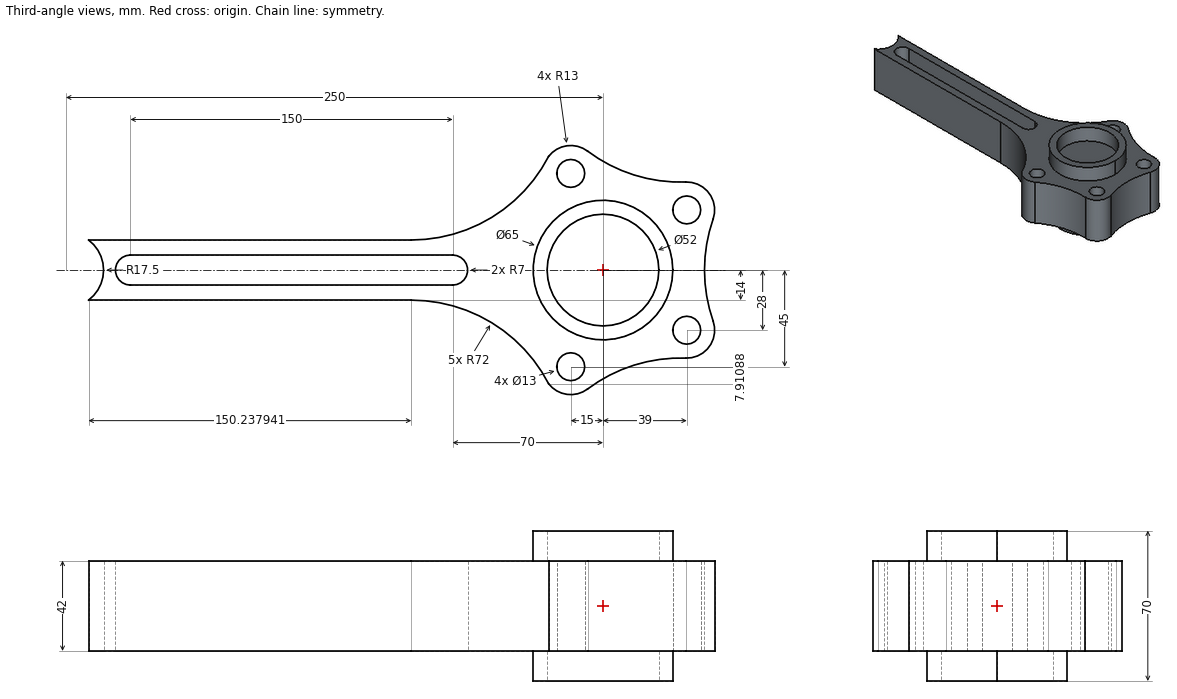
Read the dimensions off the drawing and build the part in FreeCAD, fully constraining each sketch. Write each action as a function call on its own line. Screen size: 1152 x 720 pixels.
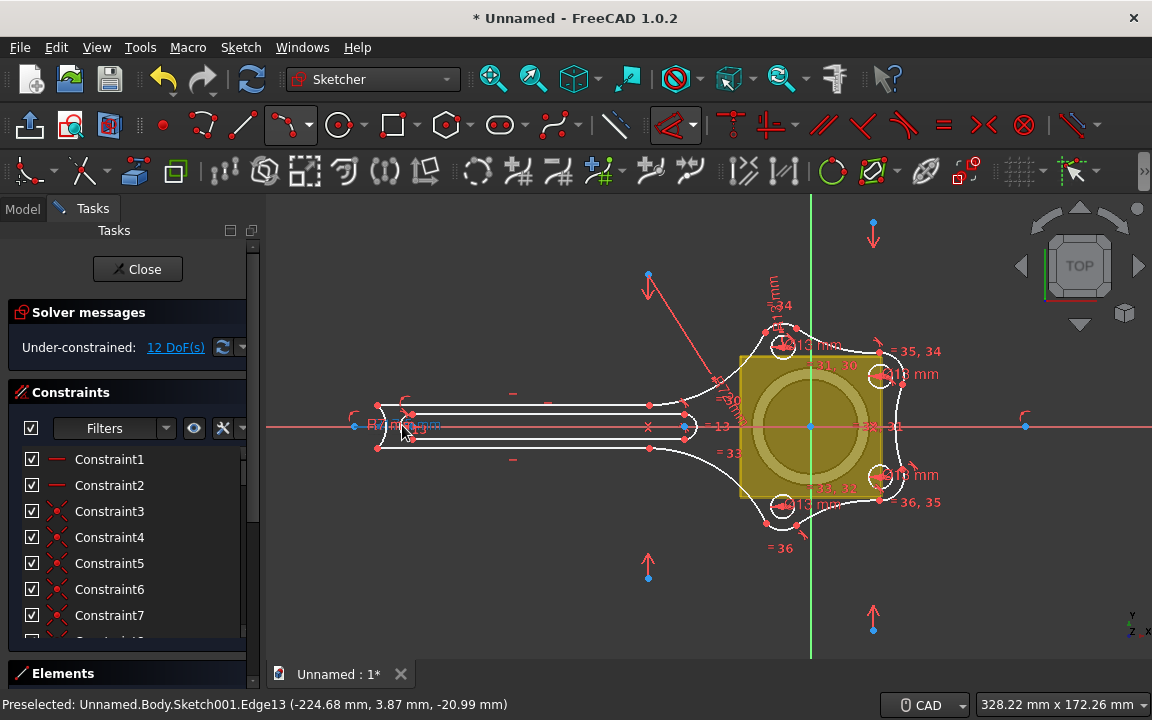
scroll(783, 507, up, 2)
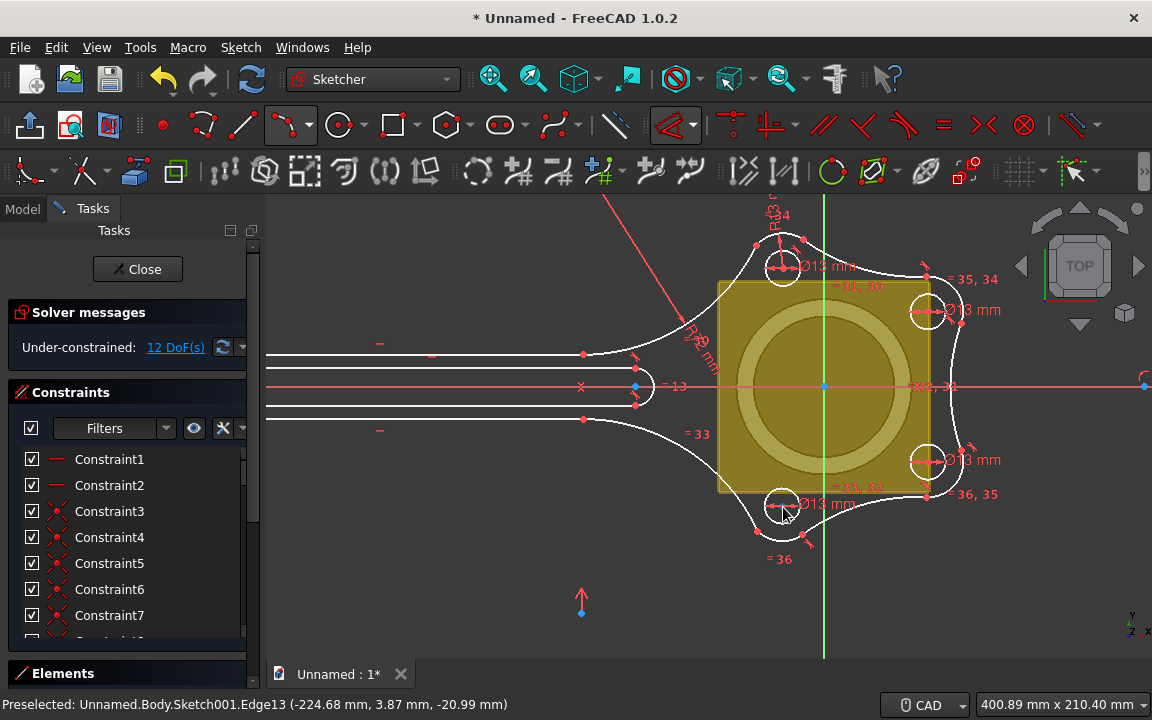
click(782, 506)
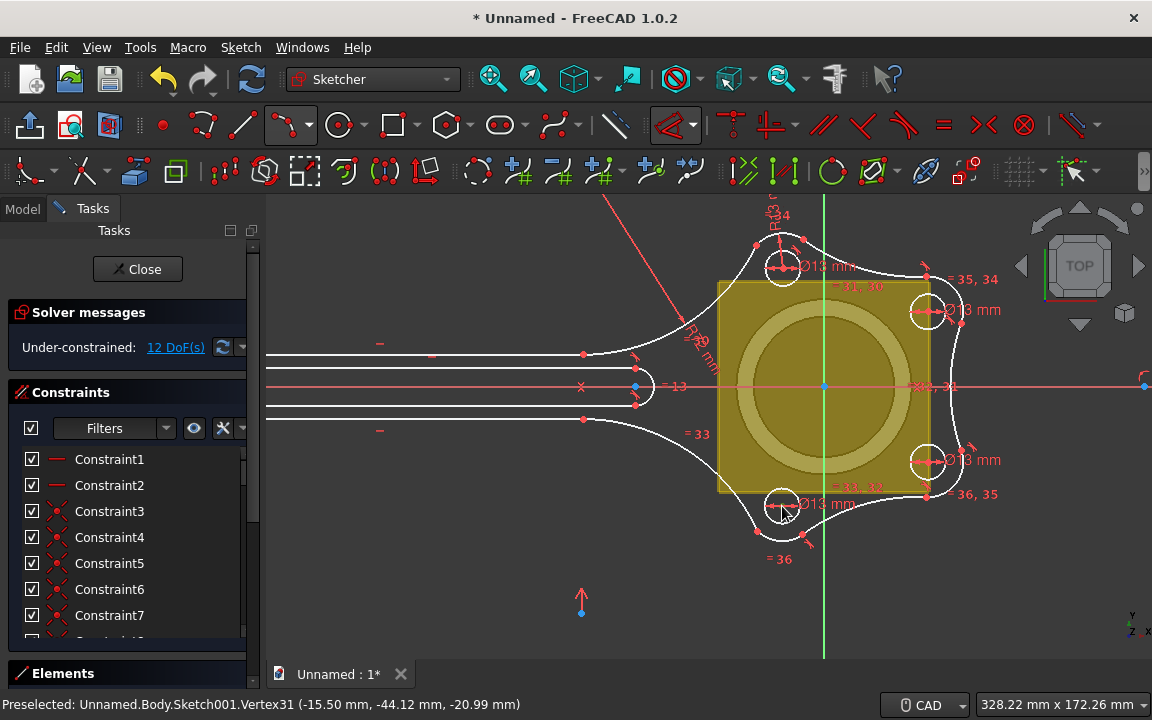
key(l)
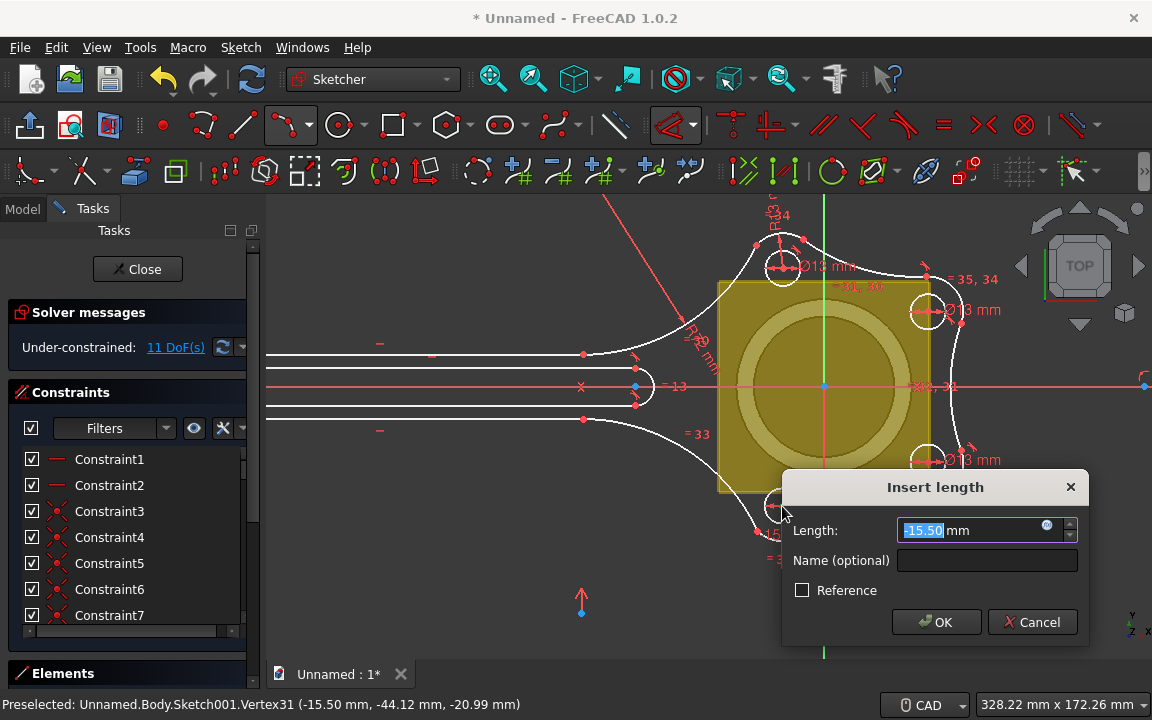
text(-15)
key(Return)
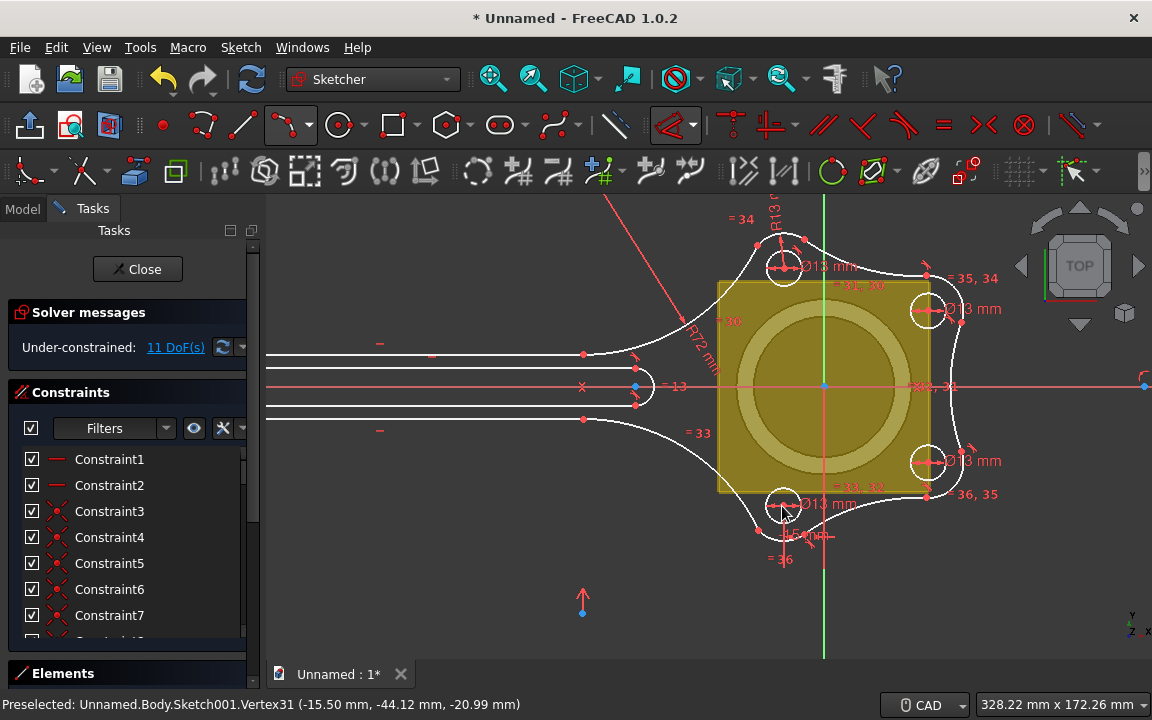
click(784, 506)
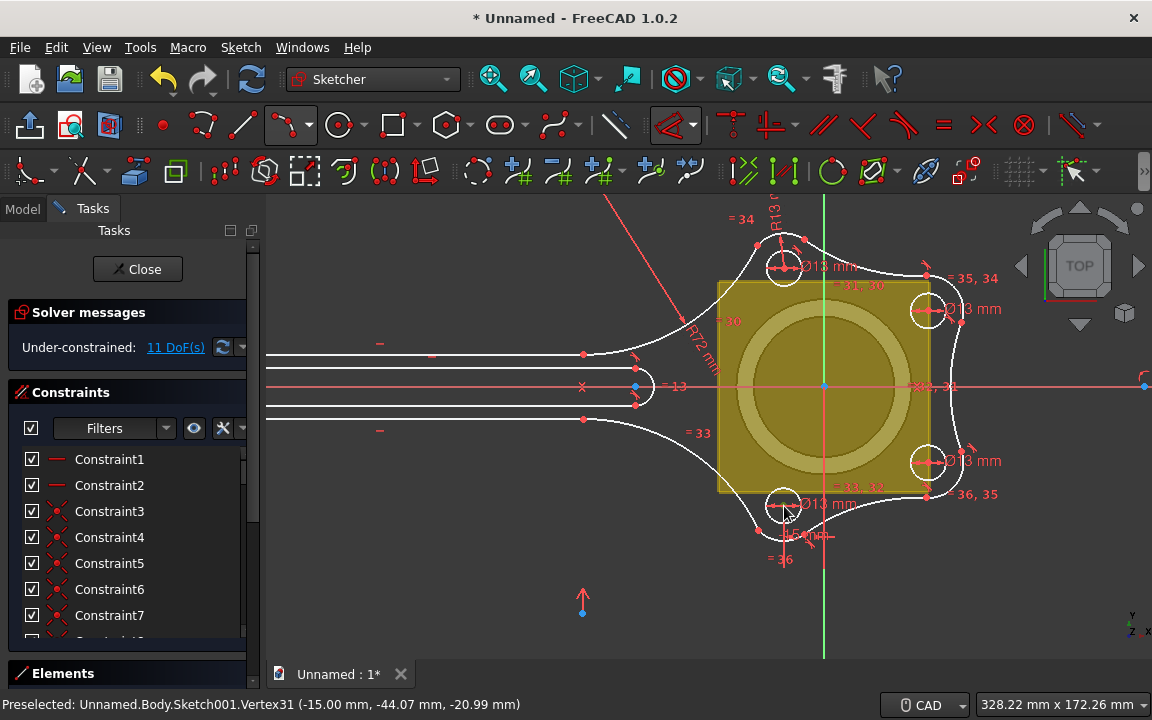
key(i)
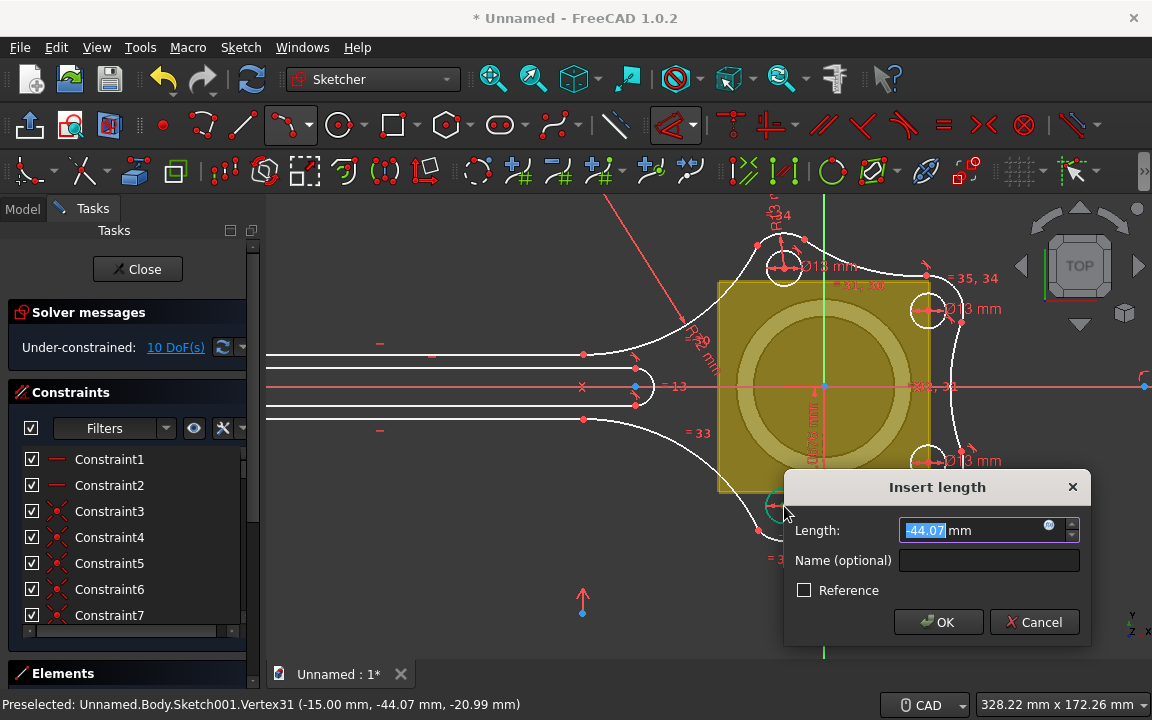
text(-45)
key(Return)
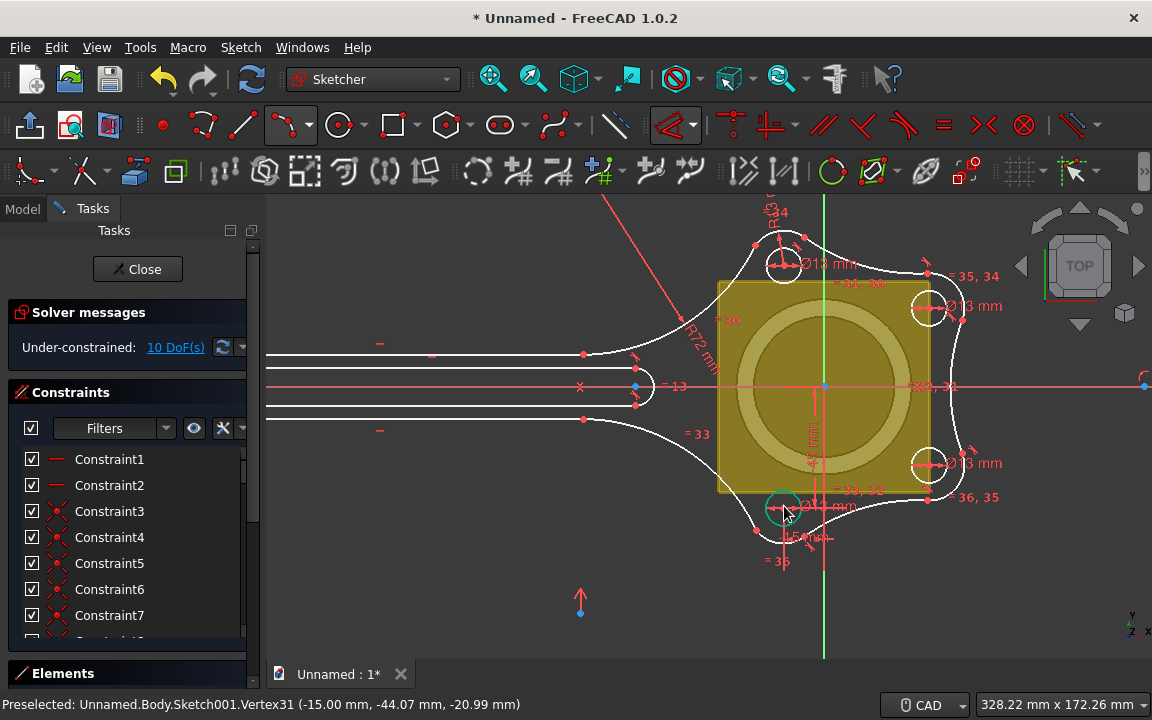
click(929, 465)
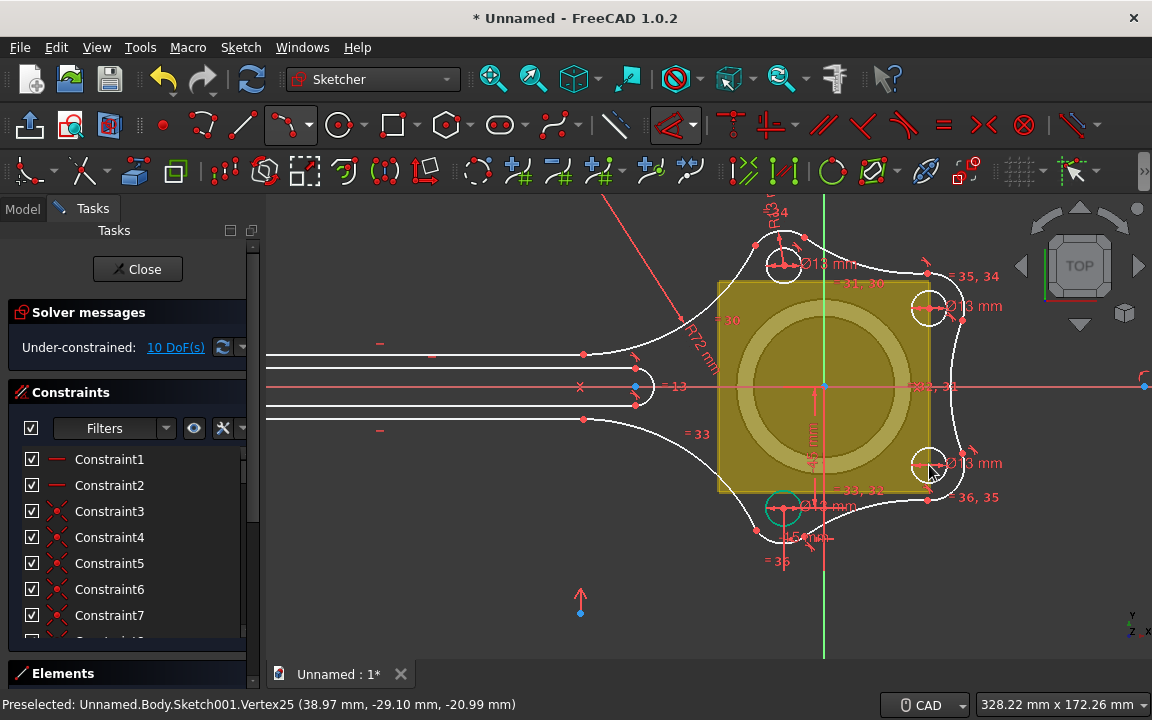
click(696, 126)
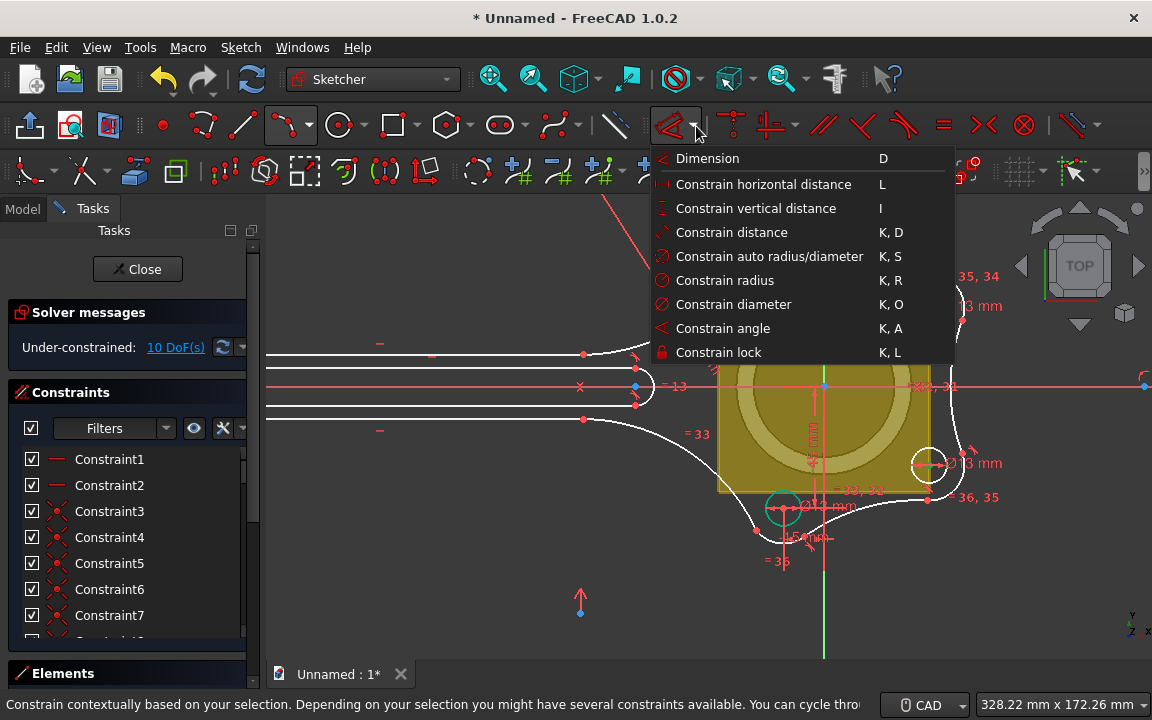
click(803, 184)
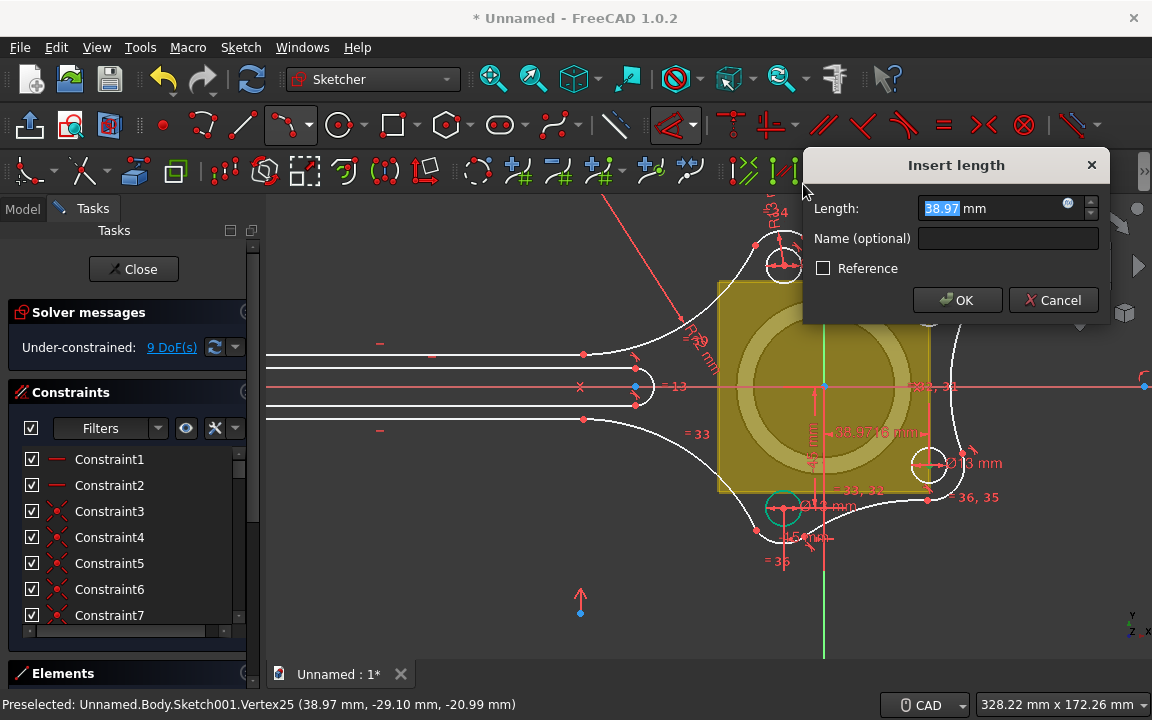
text(39)
key(Return)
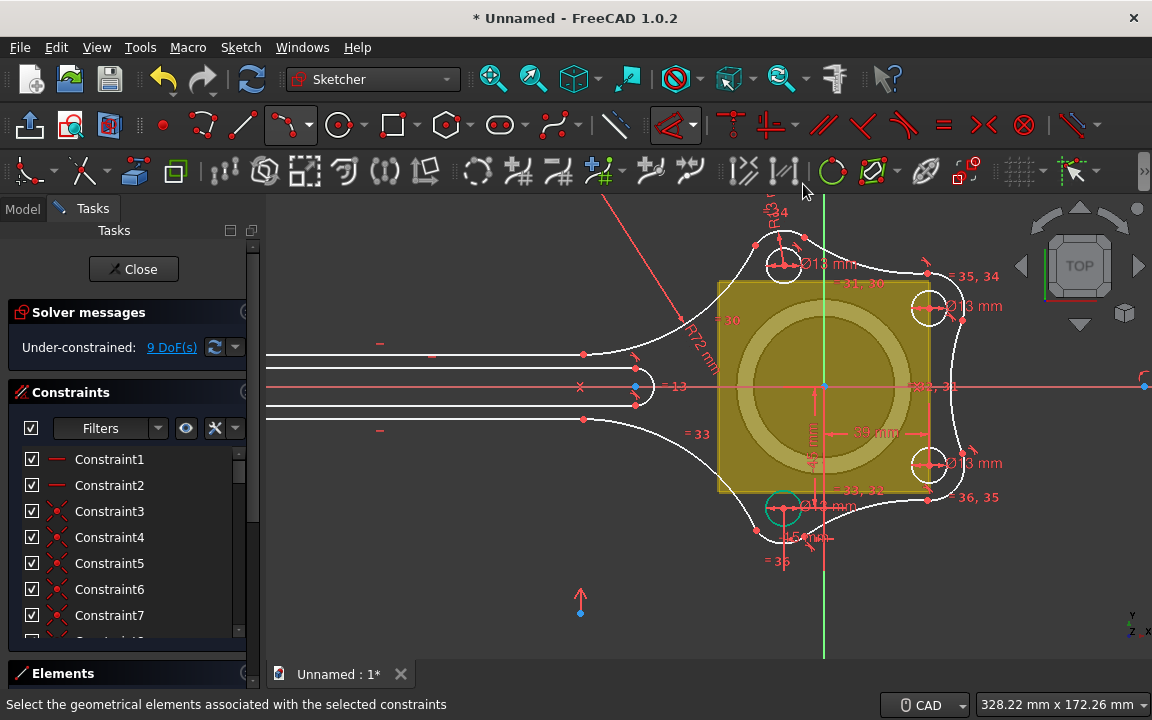
click(929, 465)